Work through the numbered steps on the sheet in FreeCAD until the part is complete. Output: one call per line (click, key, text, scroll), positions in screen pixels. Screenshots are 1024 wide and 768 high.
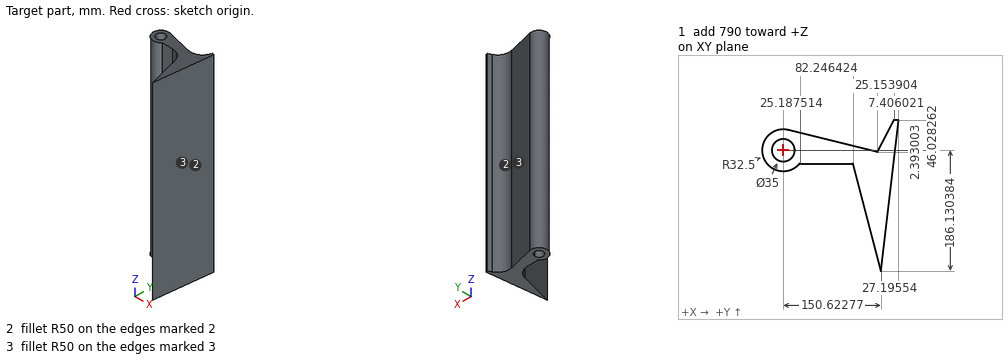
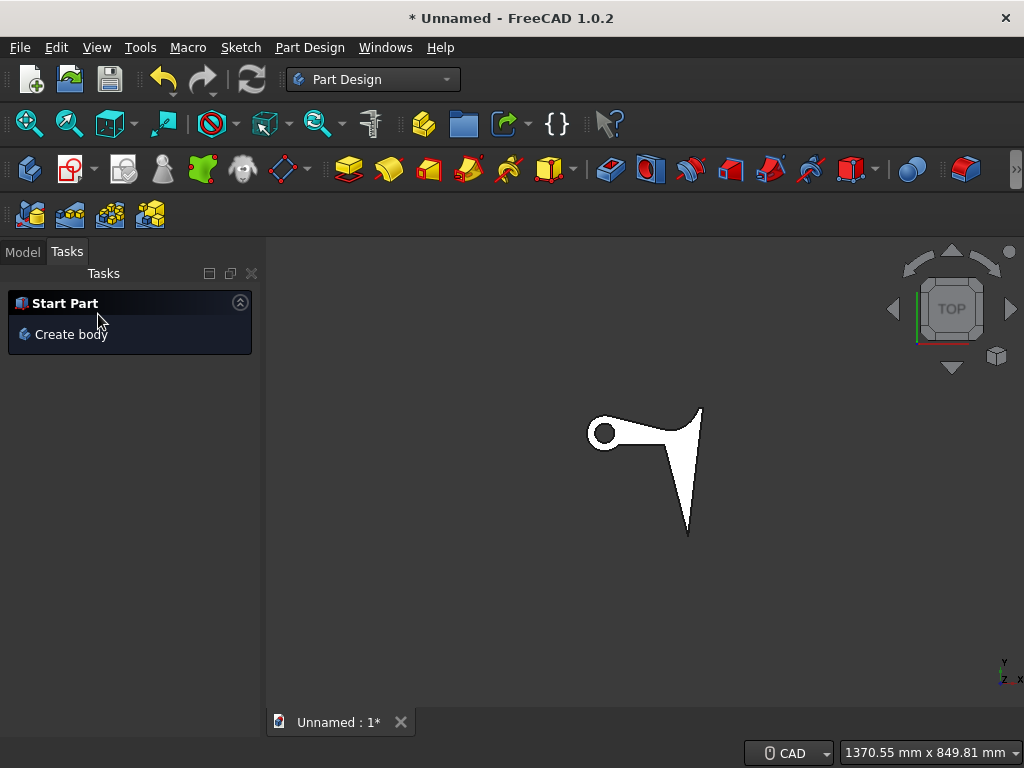
key(0)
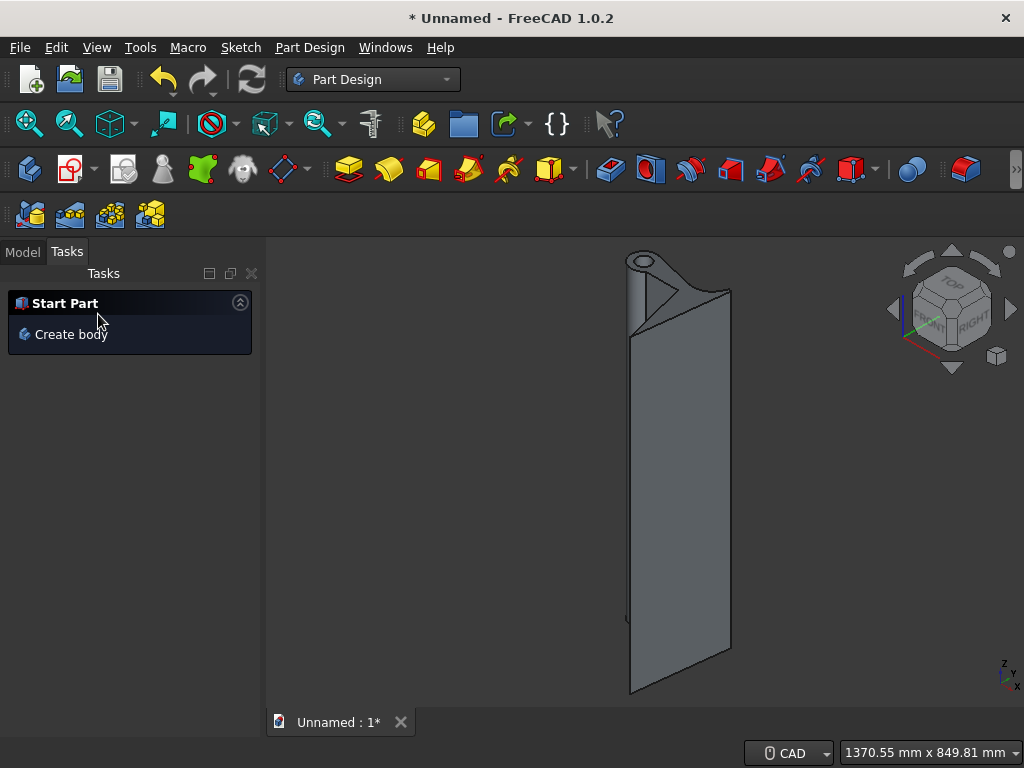
key(1)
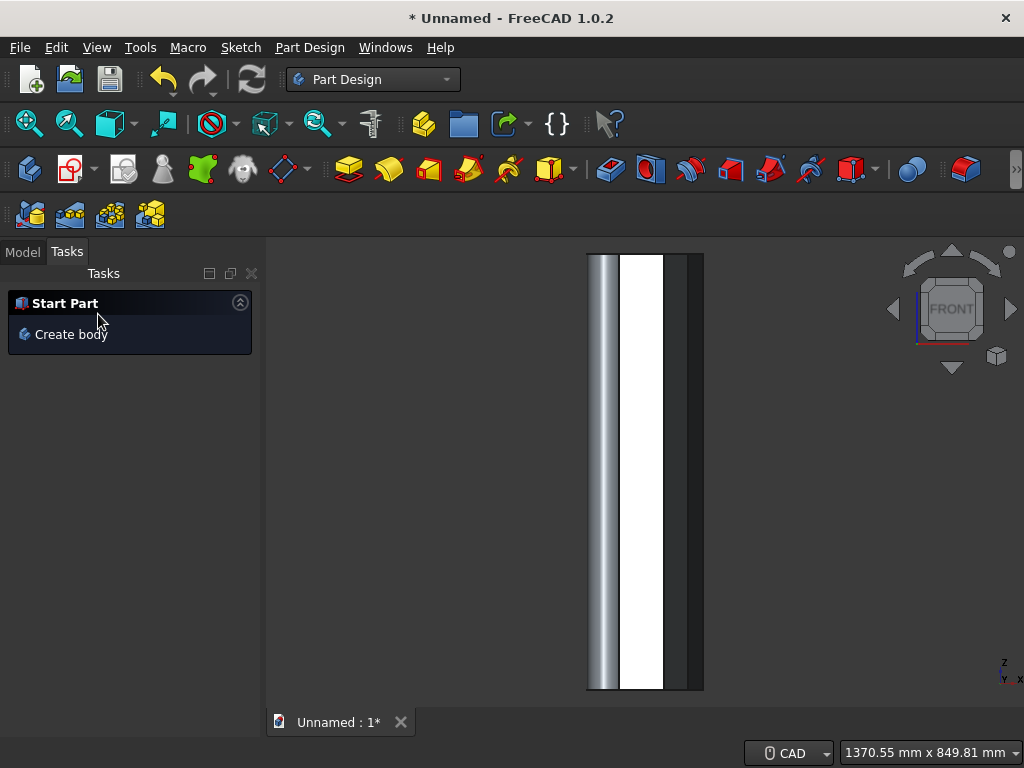
key(3)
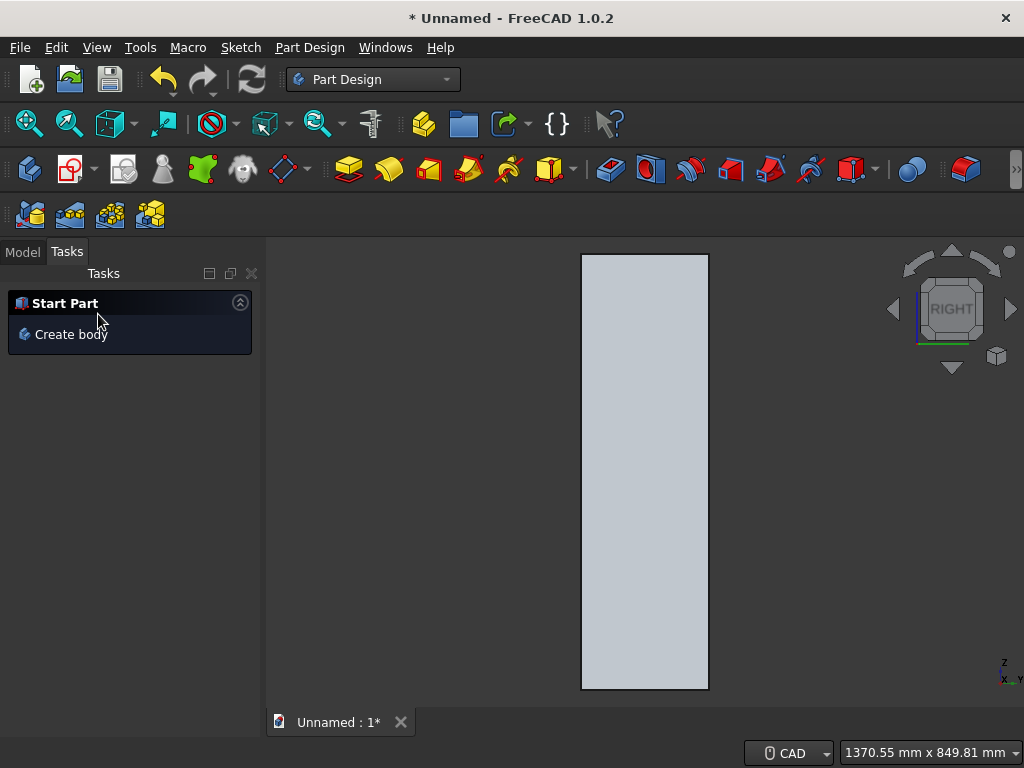
key(5)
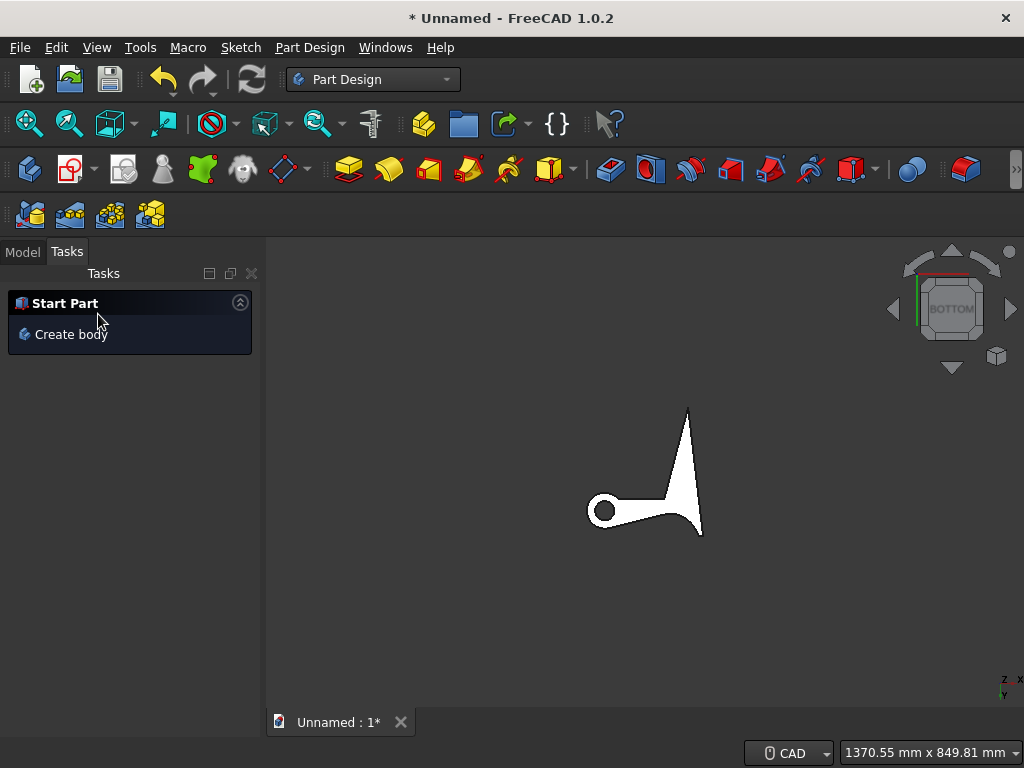
key(v)
key(f)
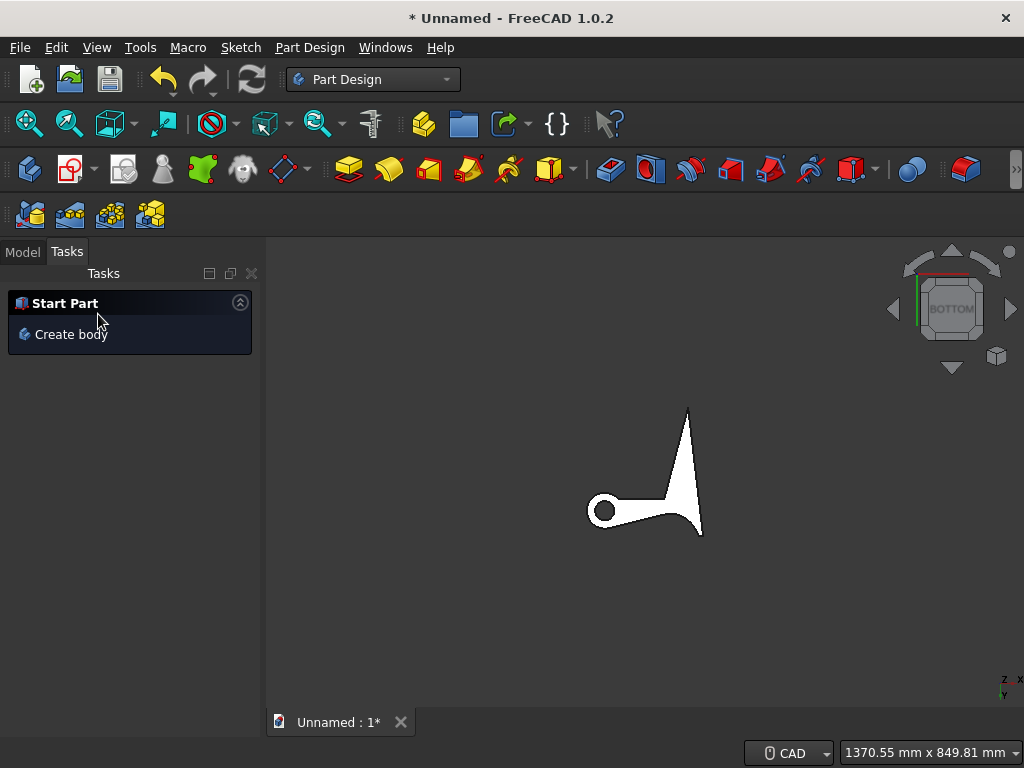
key(4)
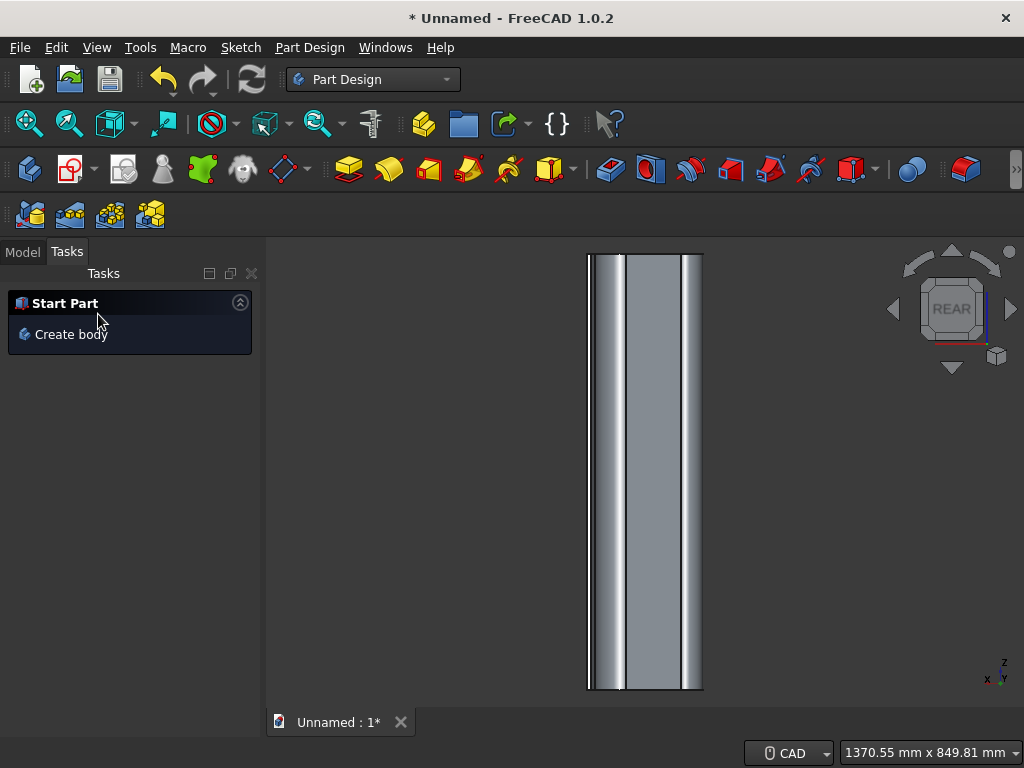
key(6)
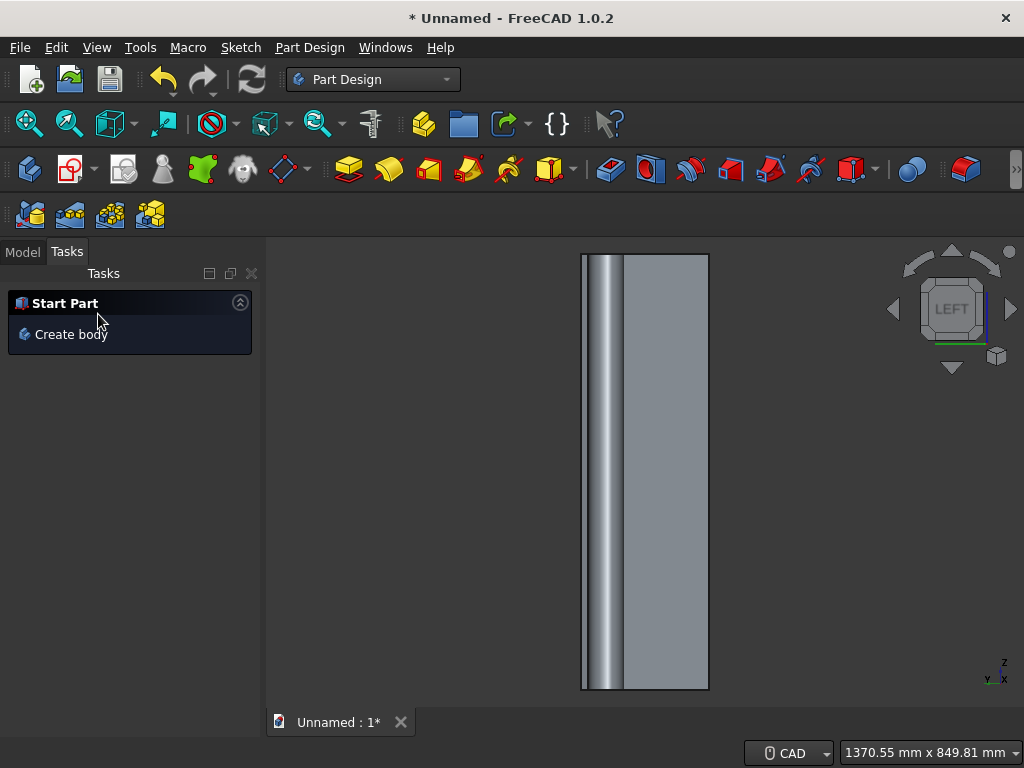
key(v)
key(3)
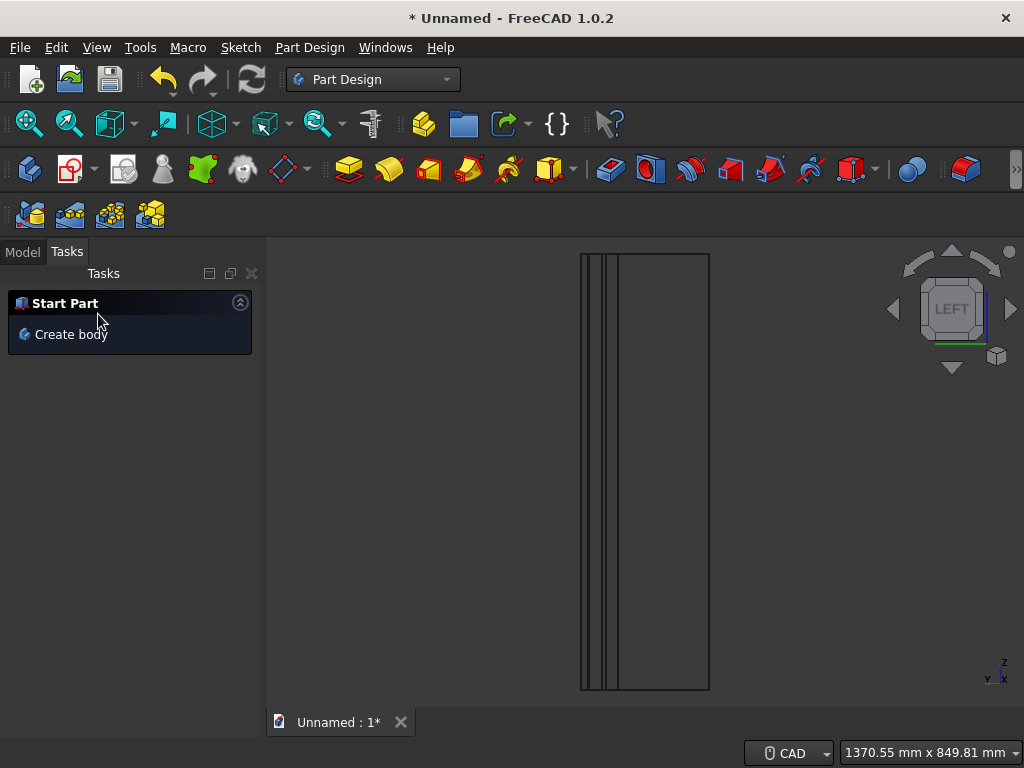
key(0)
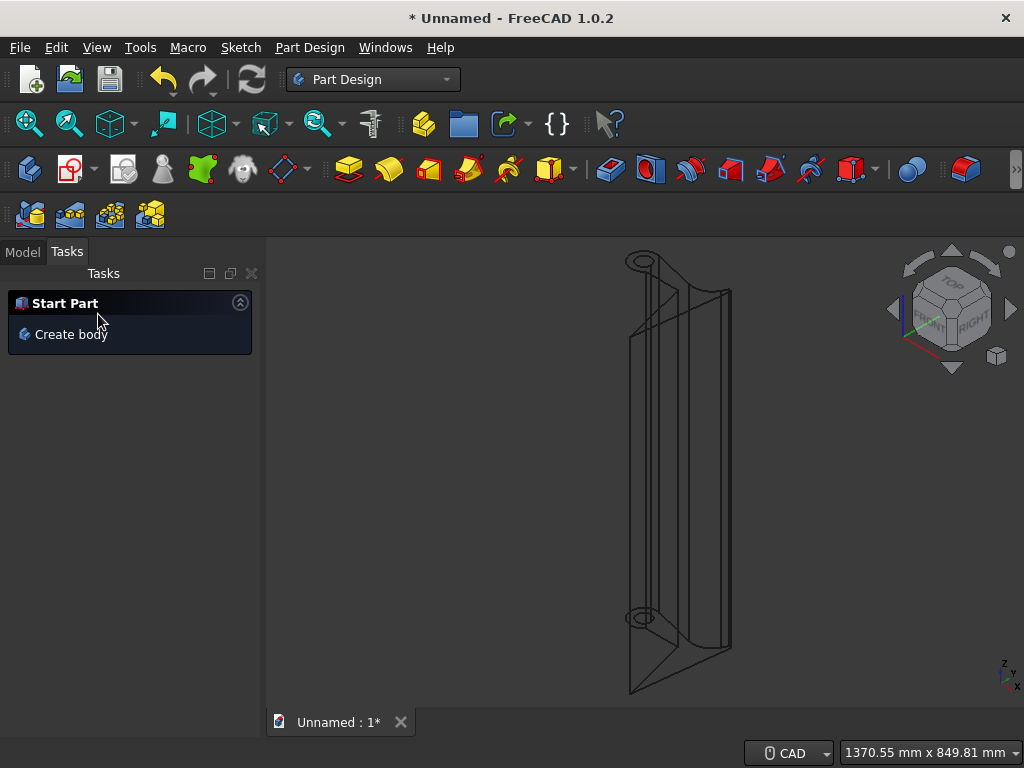
click(678, 468)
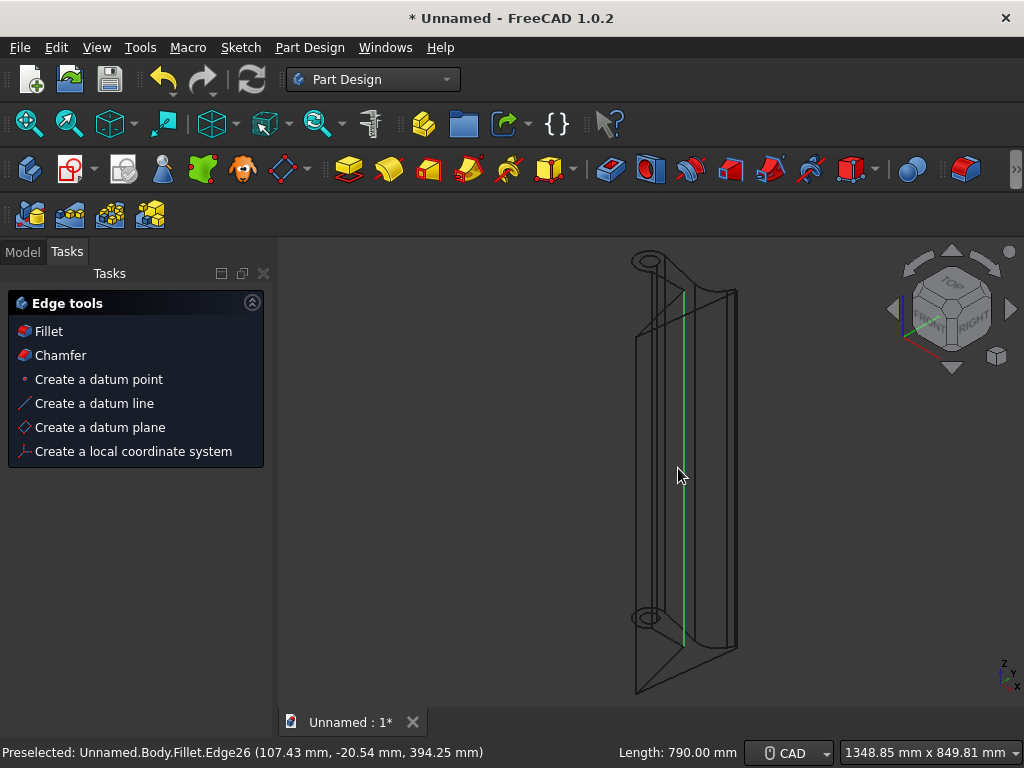
key(v)
key(1)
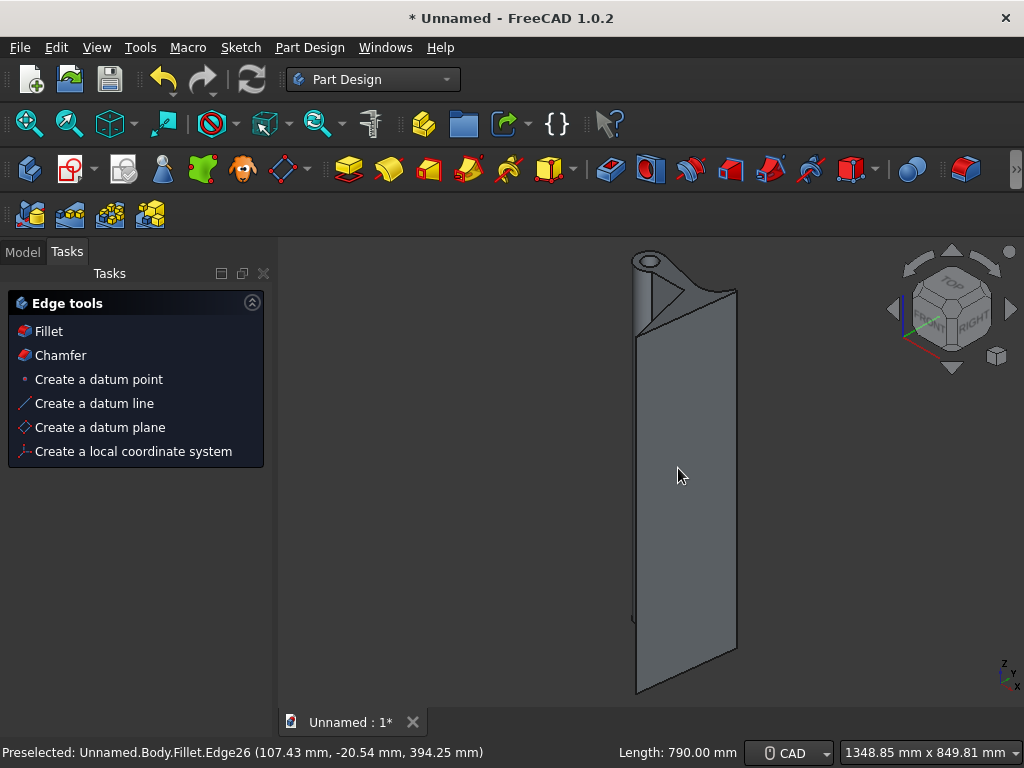
click(966, 170)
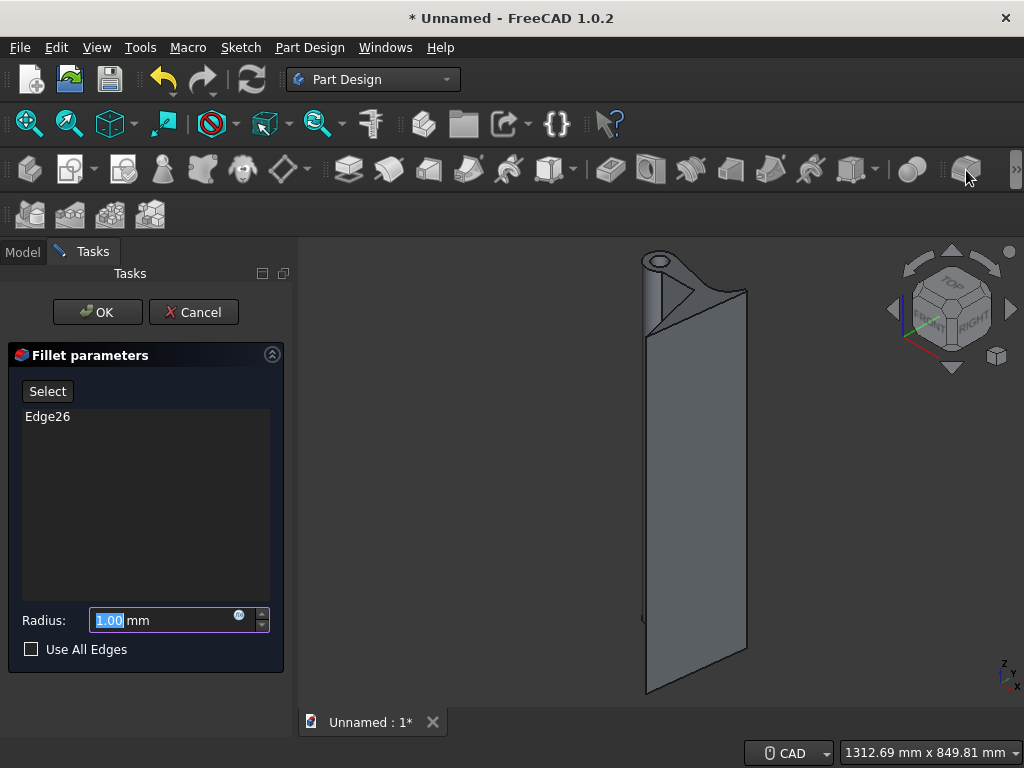
text(50)
key(Tab)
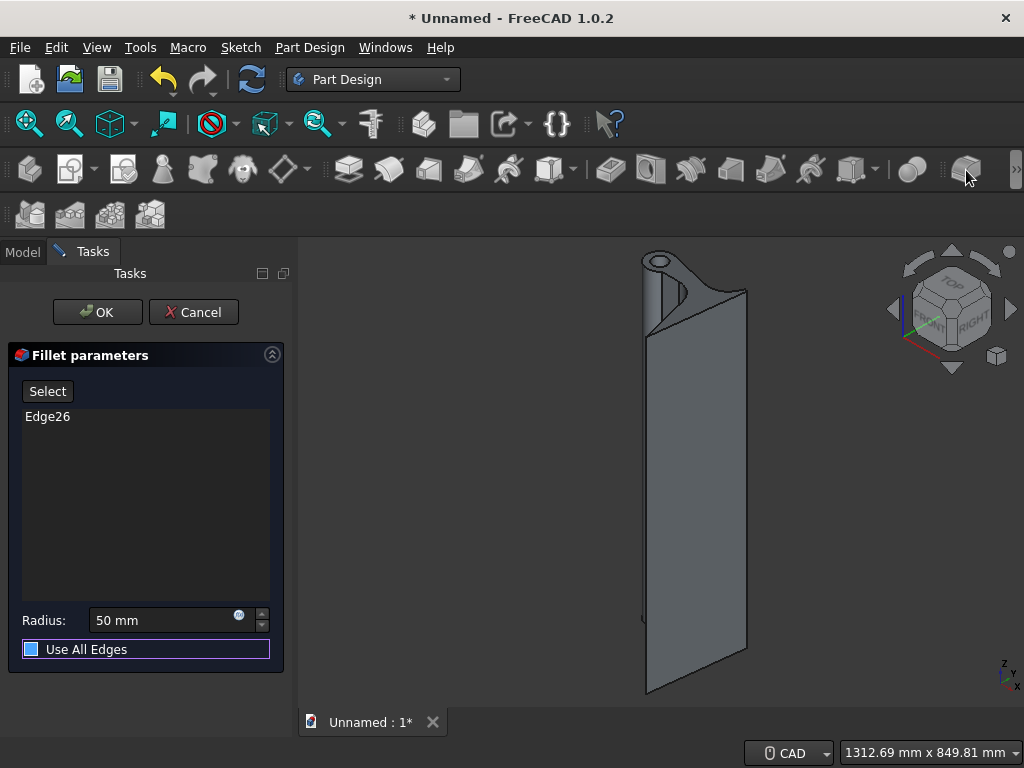
click(98, 312)